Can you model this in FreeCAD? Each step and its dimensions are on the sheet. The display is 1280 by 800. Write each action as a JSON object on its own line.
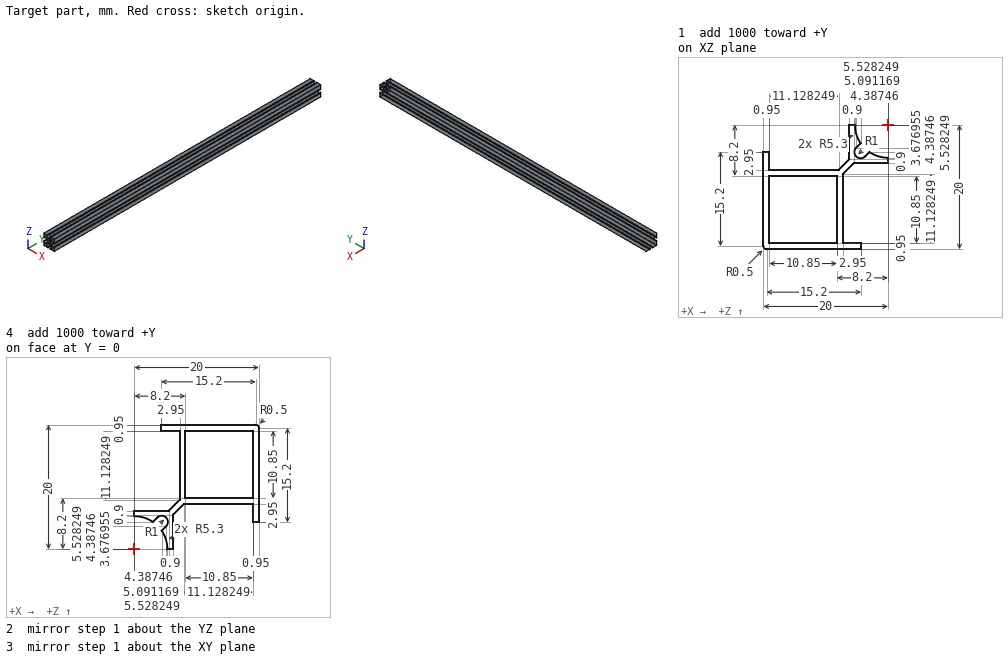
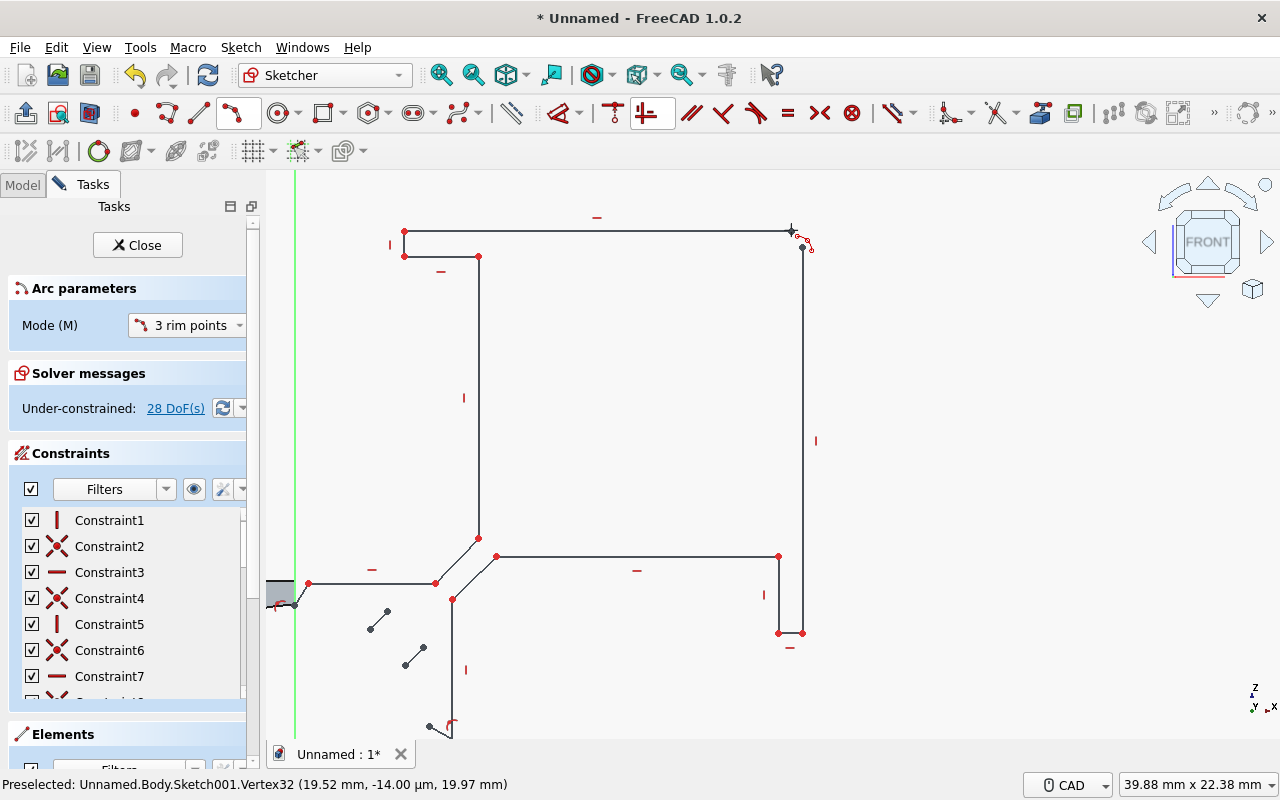
{"action": "scroll", "coordinate": [1021, 393], "scroll_direction": "down", "scroll_amount": 2}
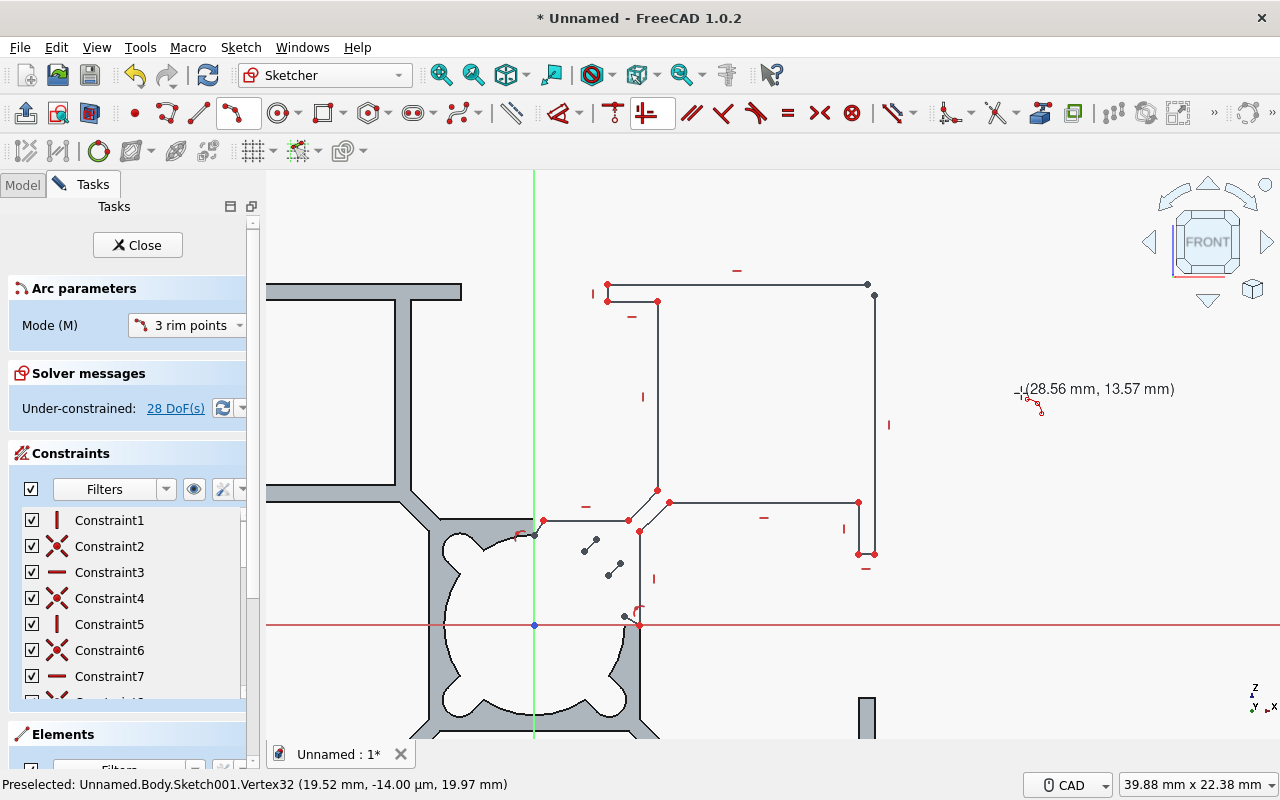
{"action": "scroll", "coordinate": [625, 625], "scroll_direction": "up", "scroll_amount": 4}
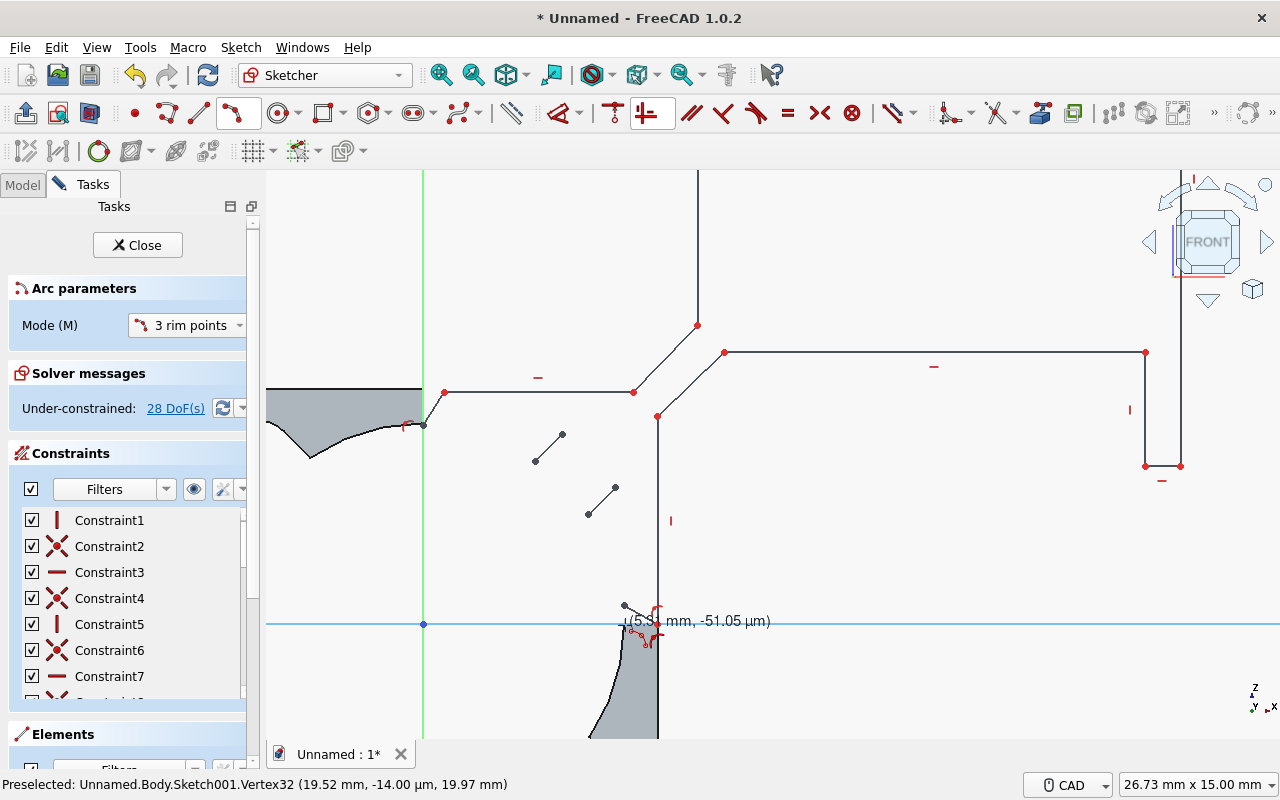
{"action": "left_click", "coordinate": [624, 606]}
{"action": "left_click", "coordinate": [589, 515]}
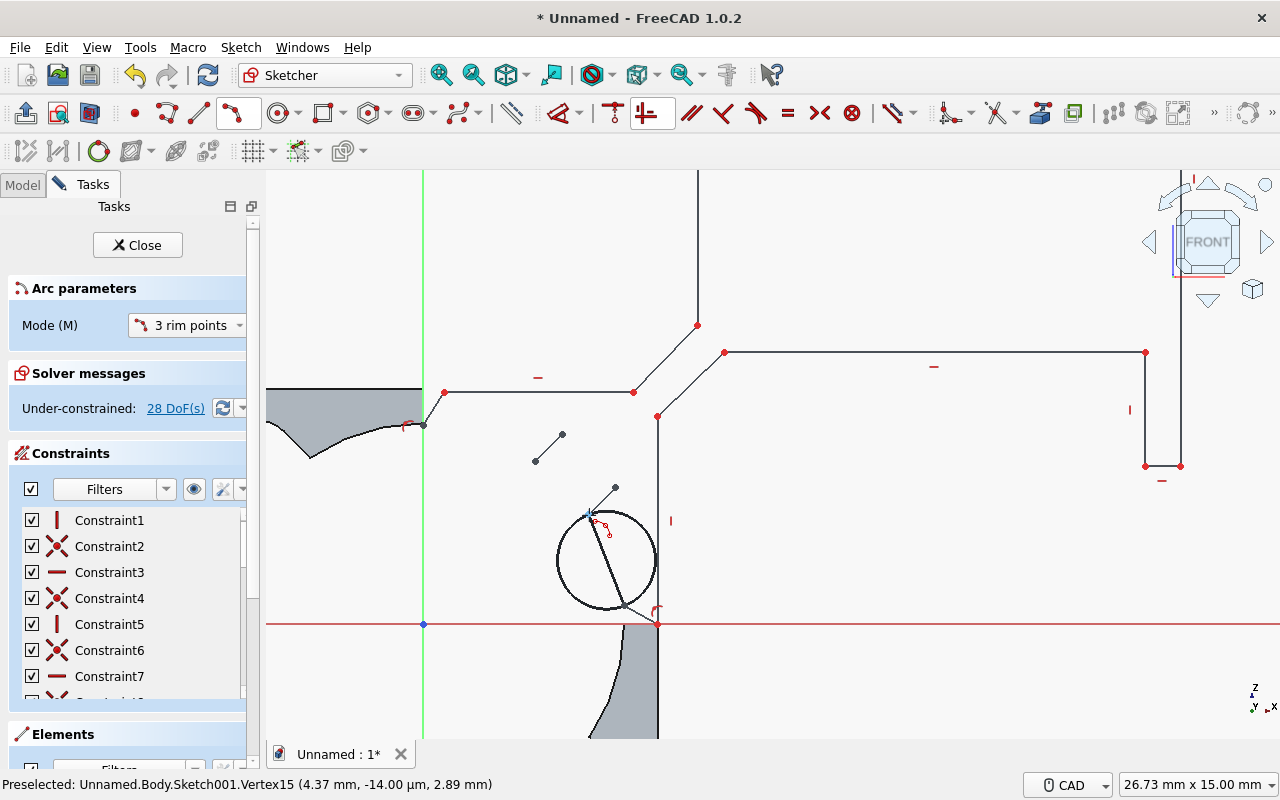
{"action": "scroll", "coordinate": [615, 565], "scroll_direction": "up", "scroll_amount": 3}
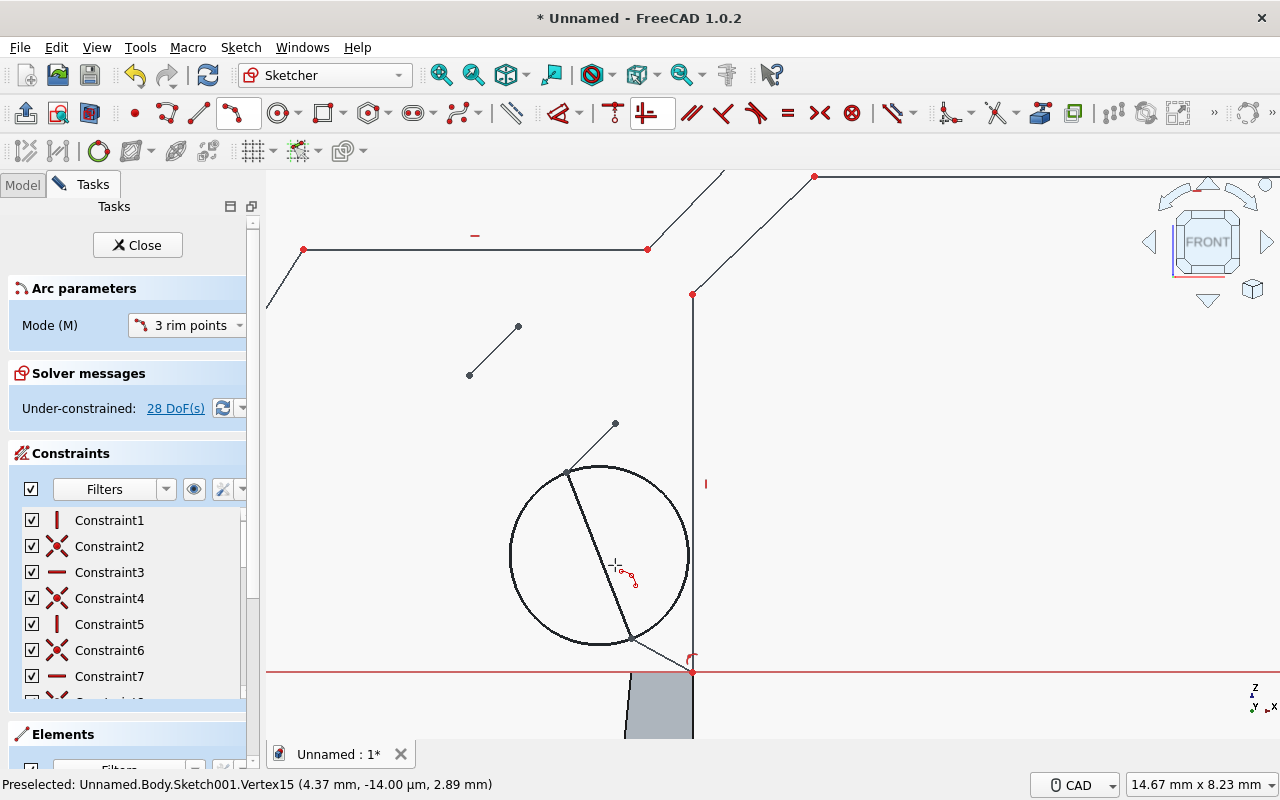
{"action": "left_click", "coordinate": [615, 565]}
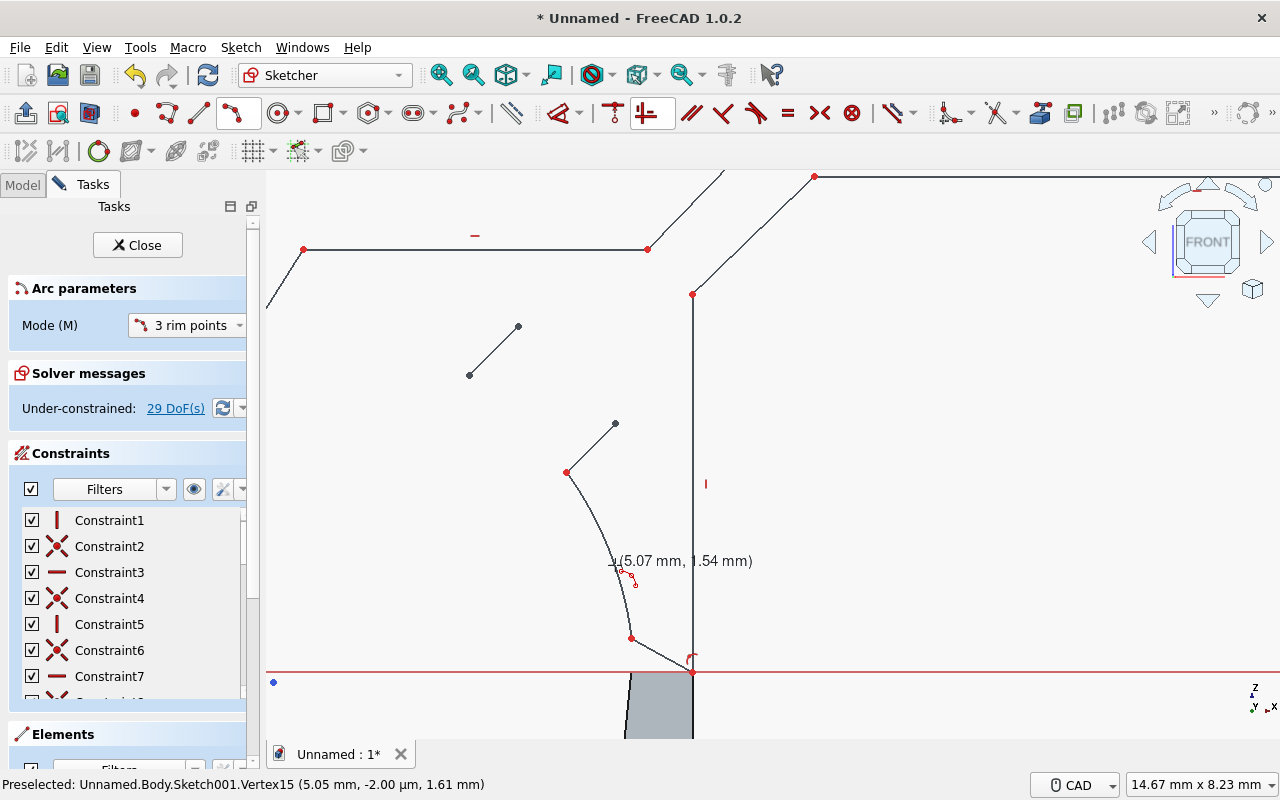
{"action": "left_click", "coordinate": [616, 424]}
{"action": "left_click", "coordinate": [518, 327]}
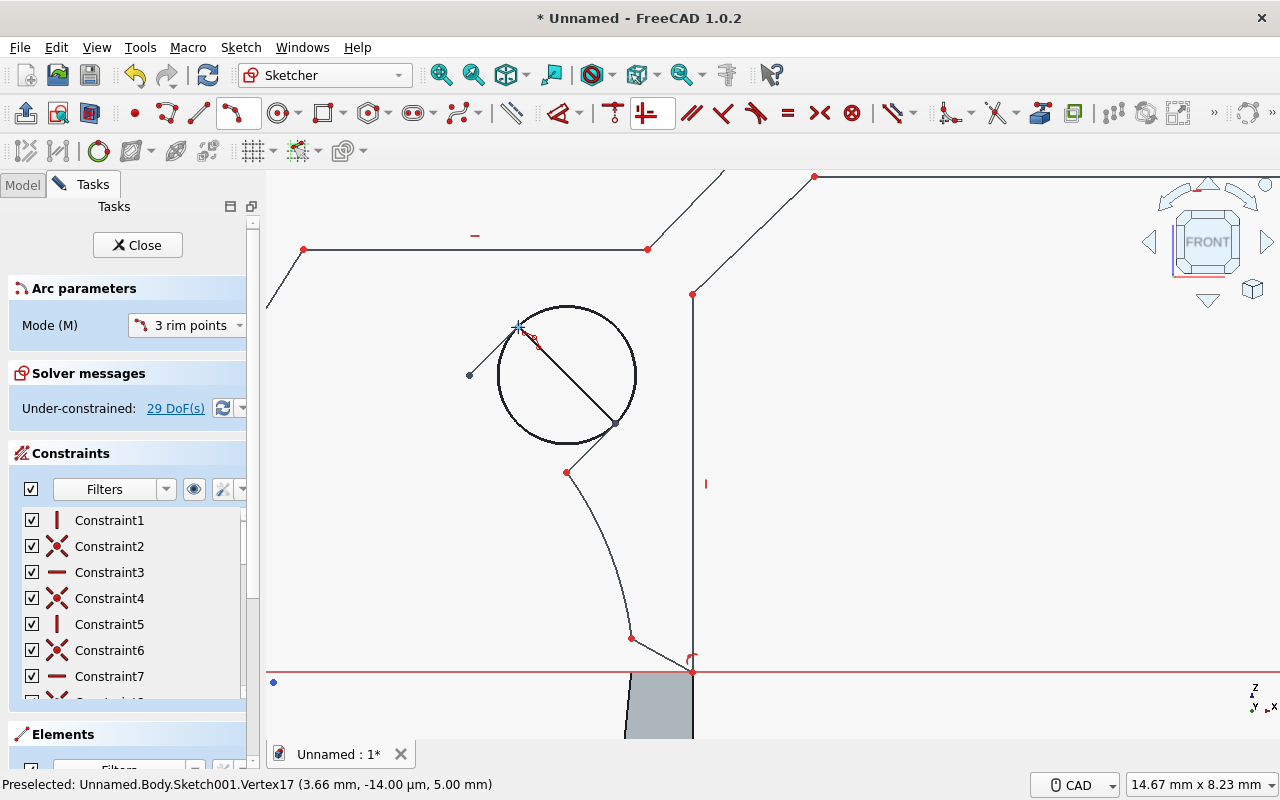
{"action": "scroll", "coordinate": [622, 609], "scroll_direction": "down", "scroll_amount": 7}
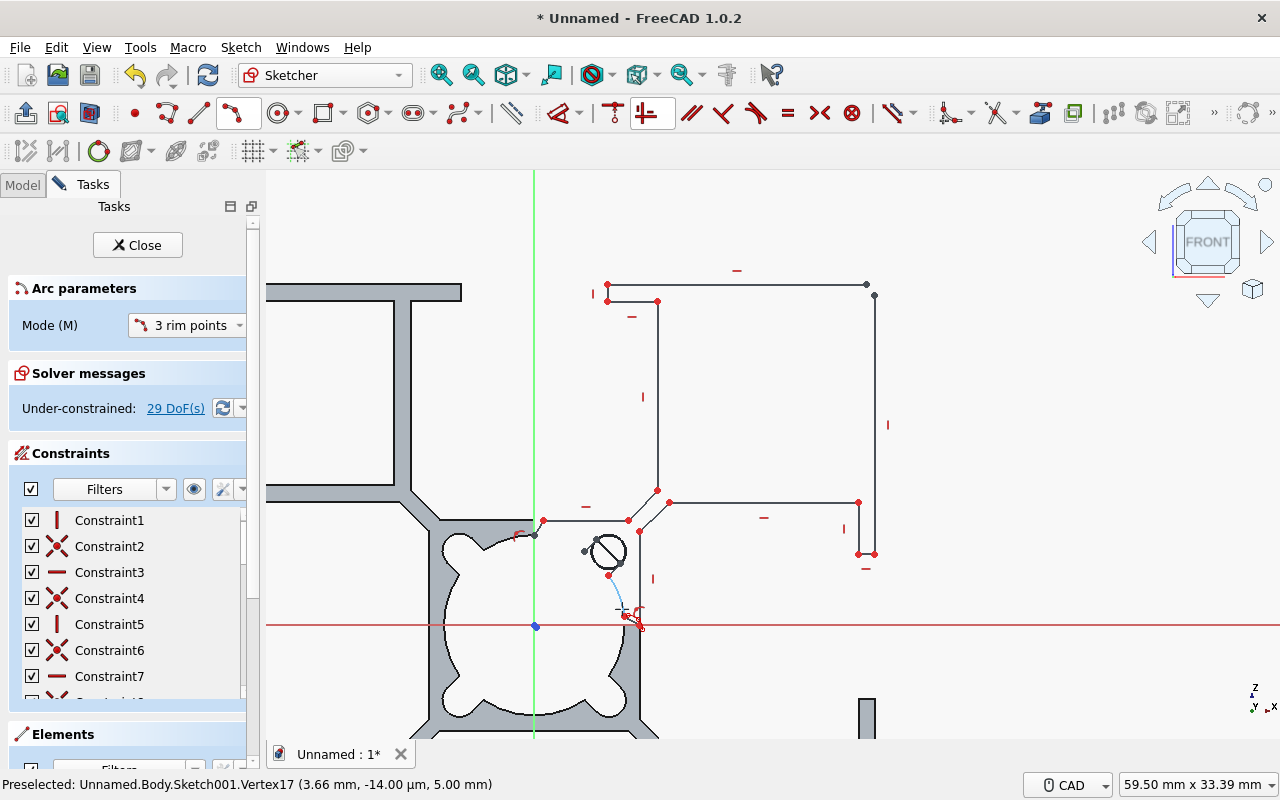
{"action": "left_click", "coordinate": [621, 538]}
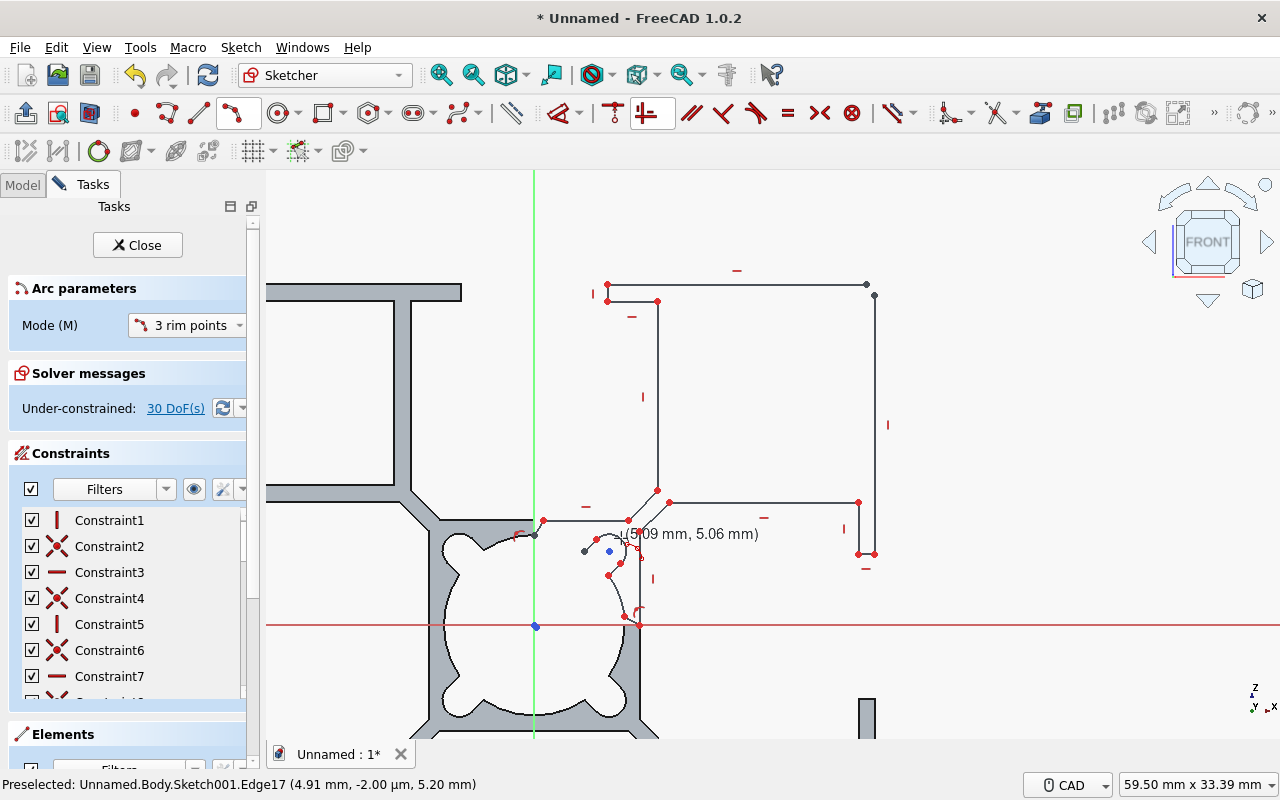
{"action": "scroll", "coordinate": [585, 550], "scroll_direction": "up", "scroll_amount": 4}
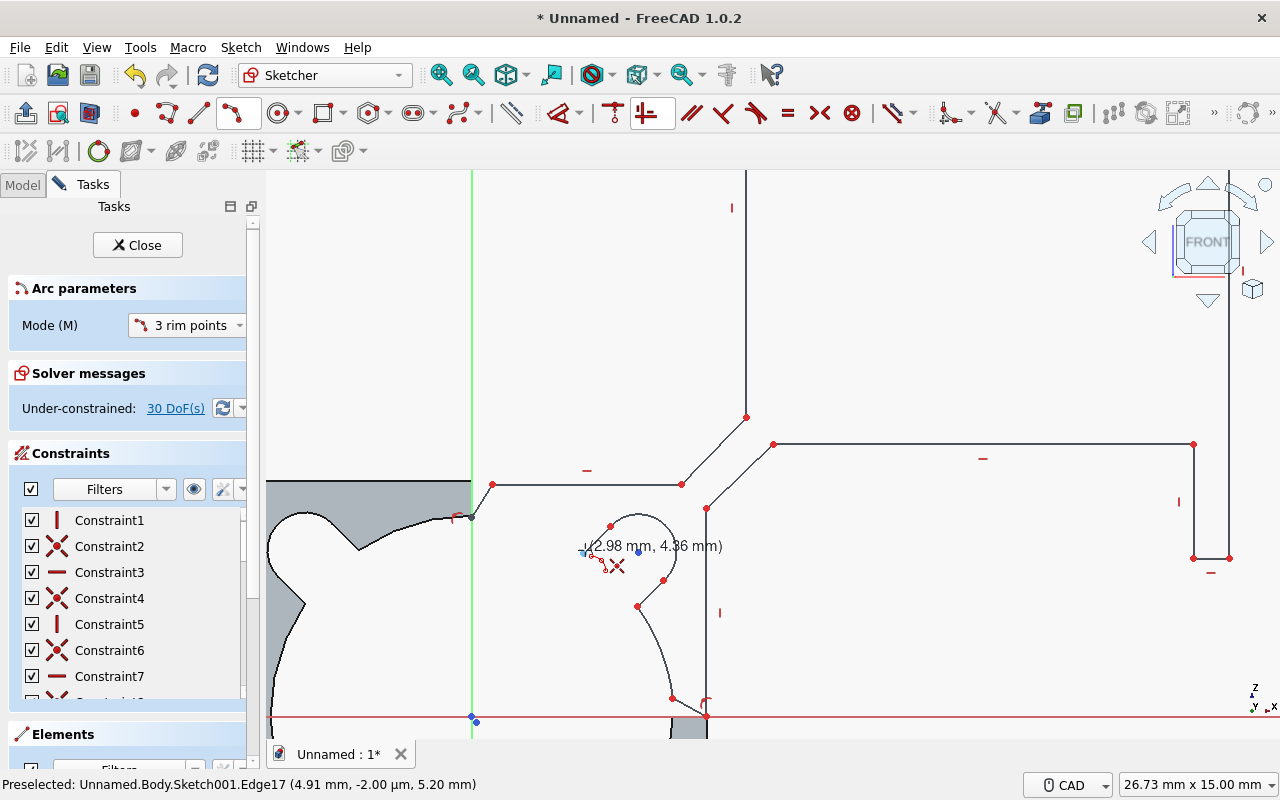
{"action": "left_click", "coordinate": [584, 554]}
{"action": "left_click", "coordinate": [472, 518]}